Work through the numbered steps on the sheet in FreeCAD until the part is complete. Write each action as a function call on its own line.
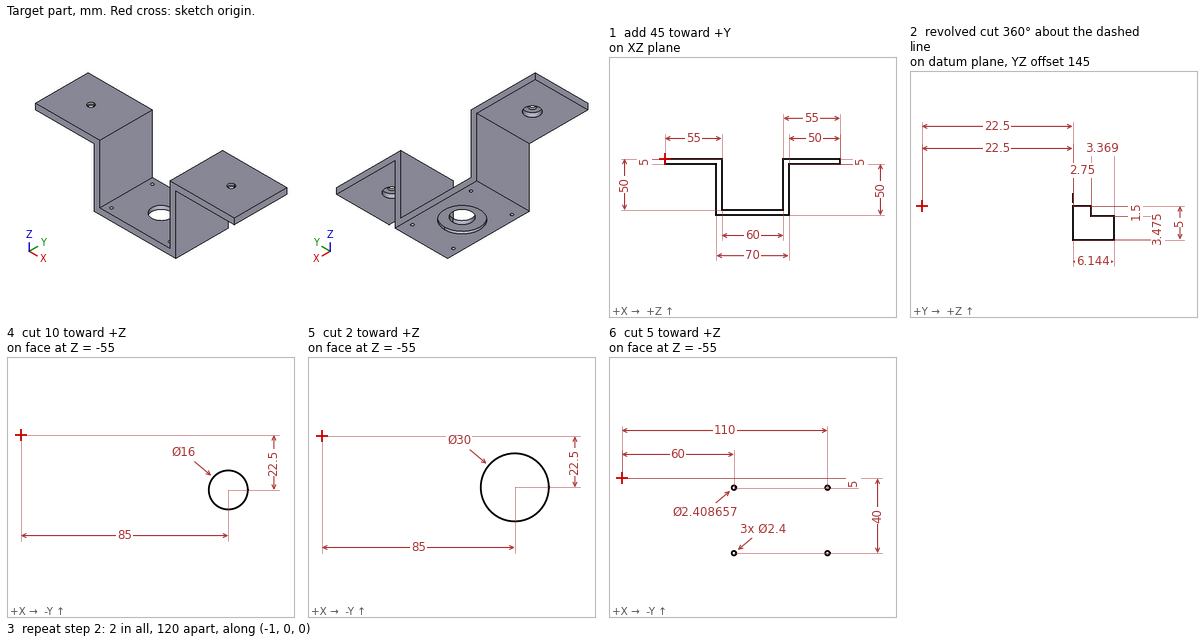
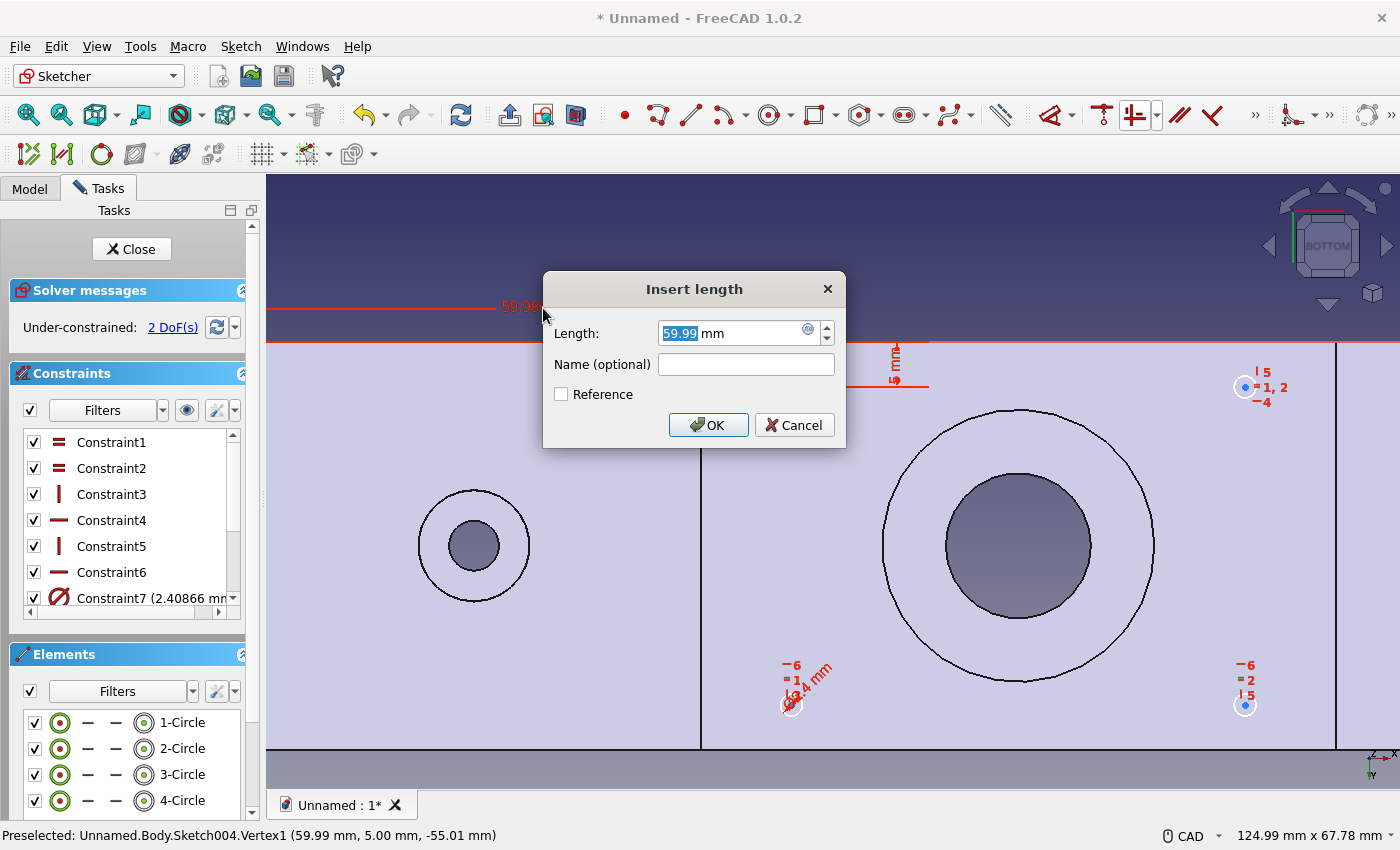
text(60)
key(Return)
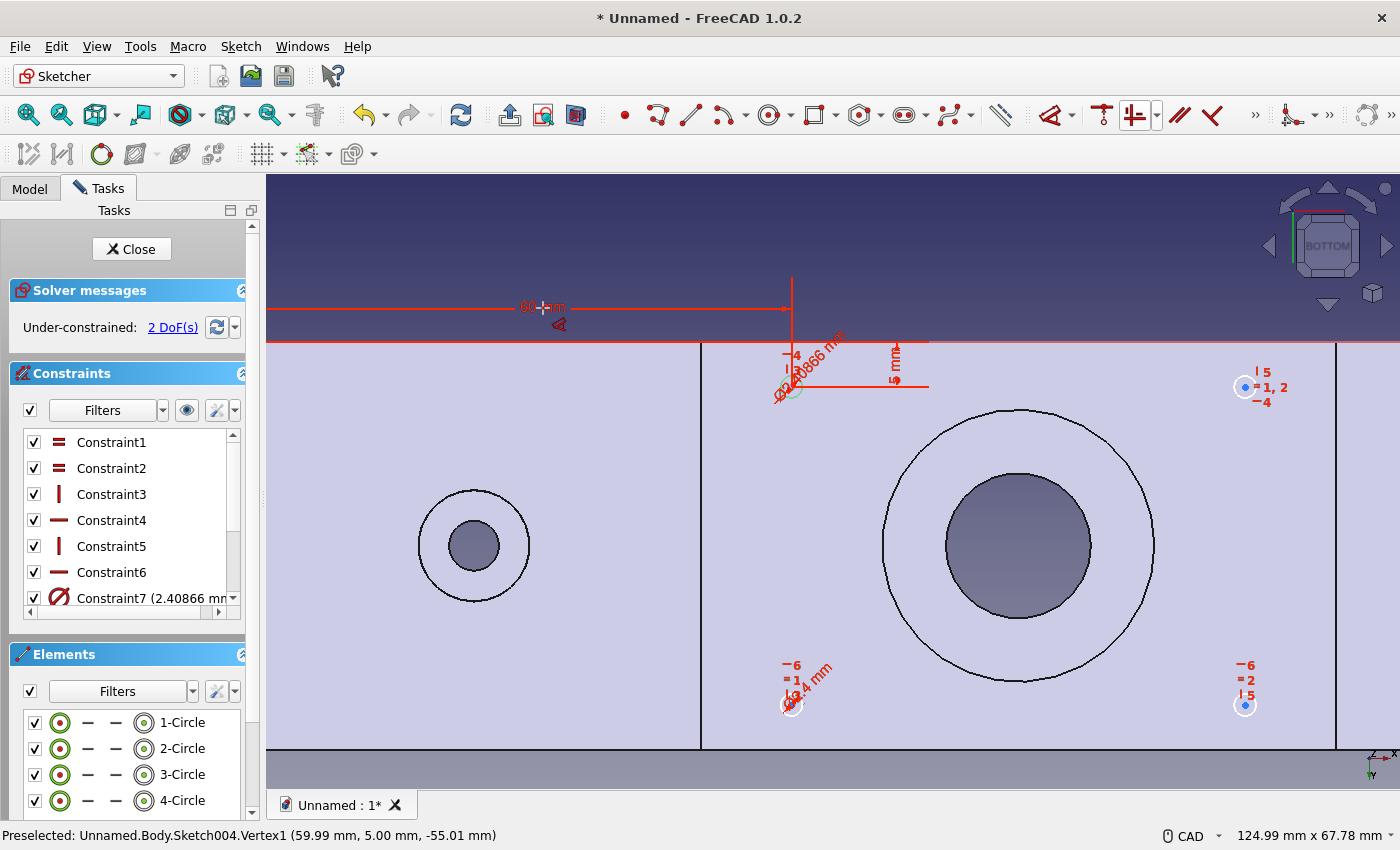
click(792, 705)
click(826, 523)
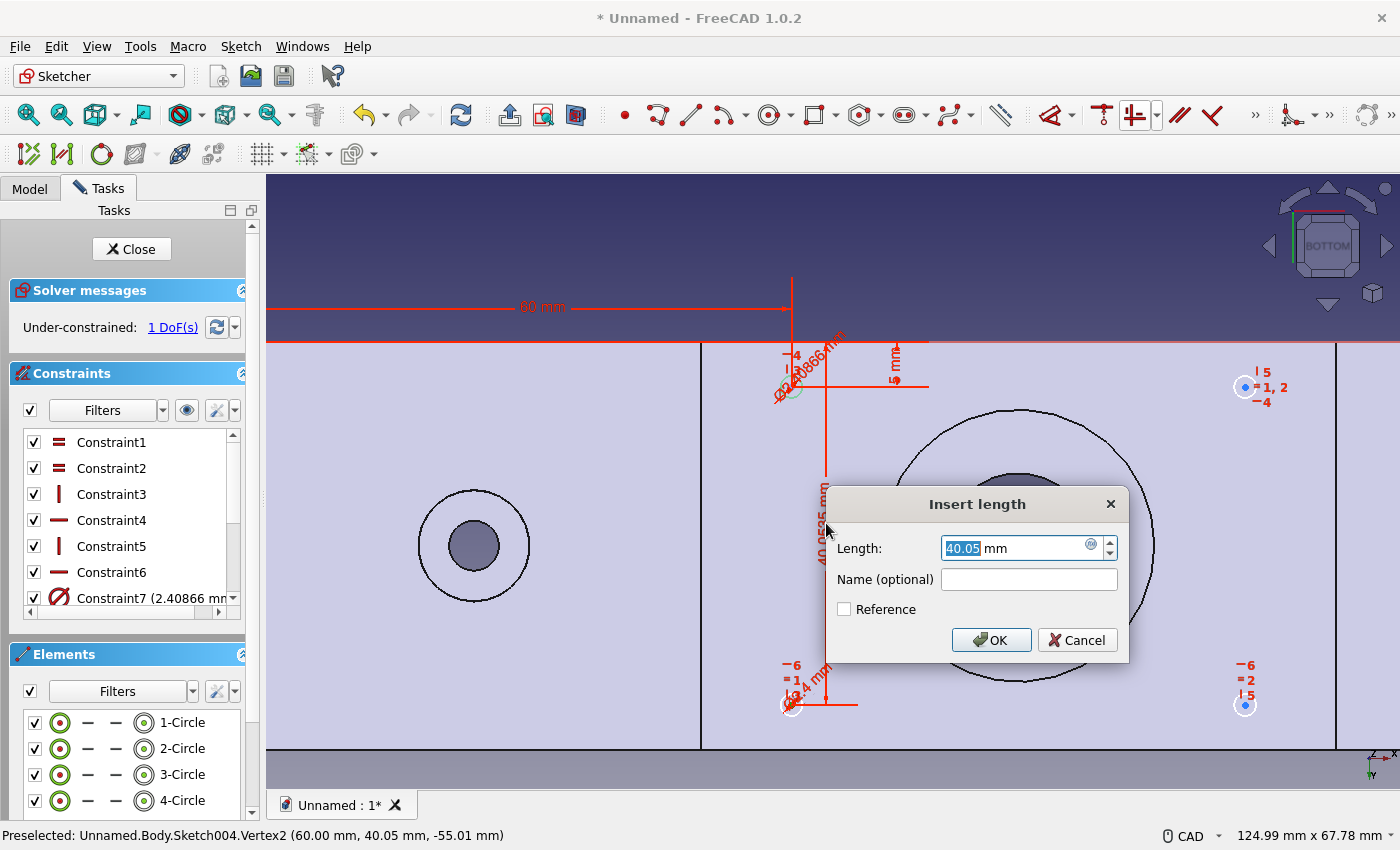
text(40)
key(Return)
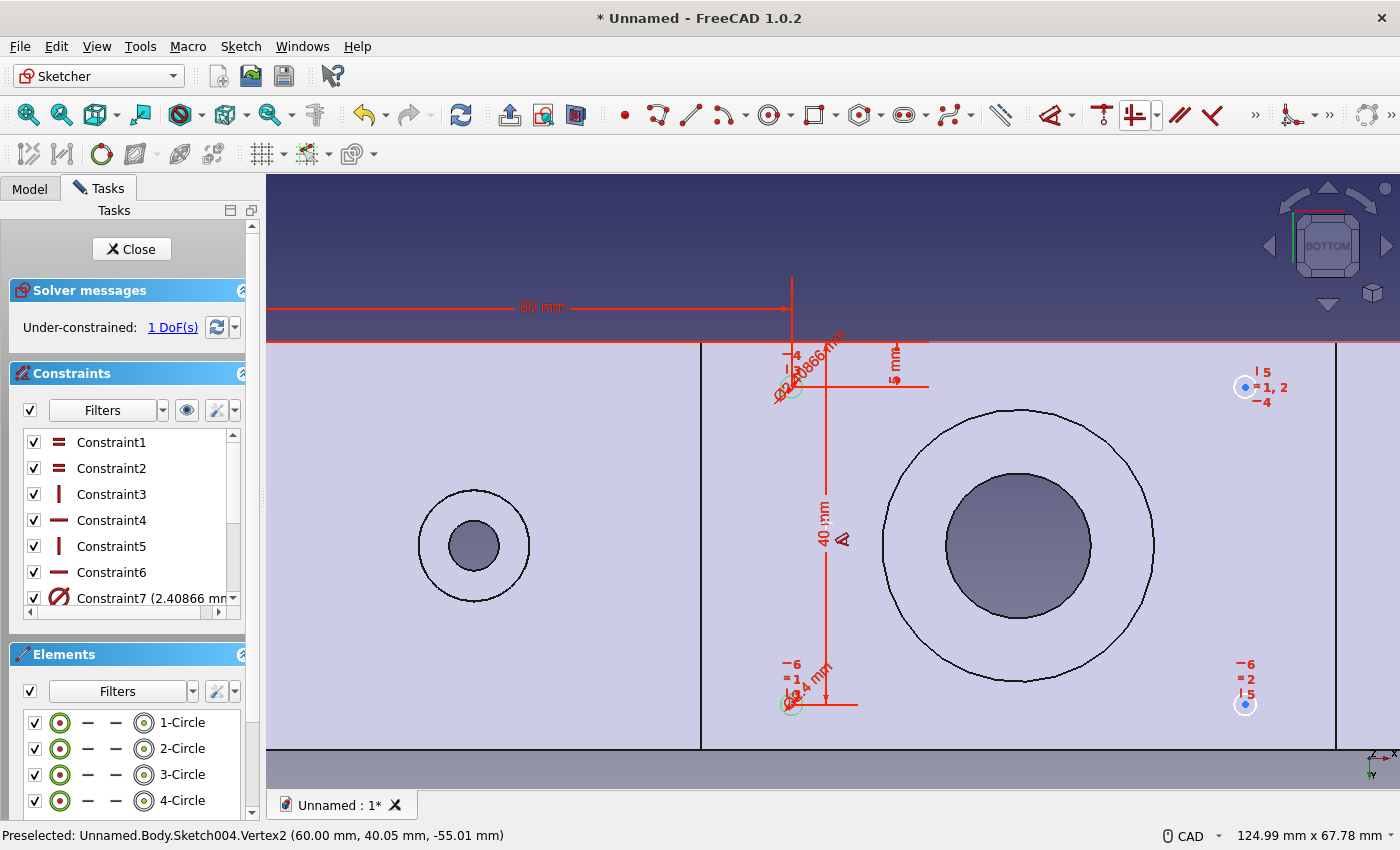
scroll(791, 386, down, 2)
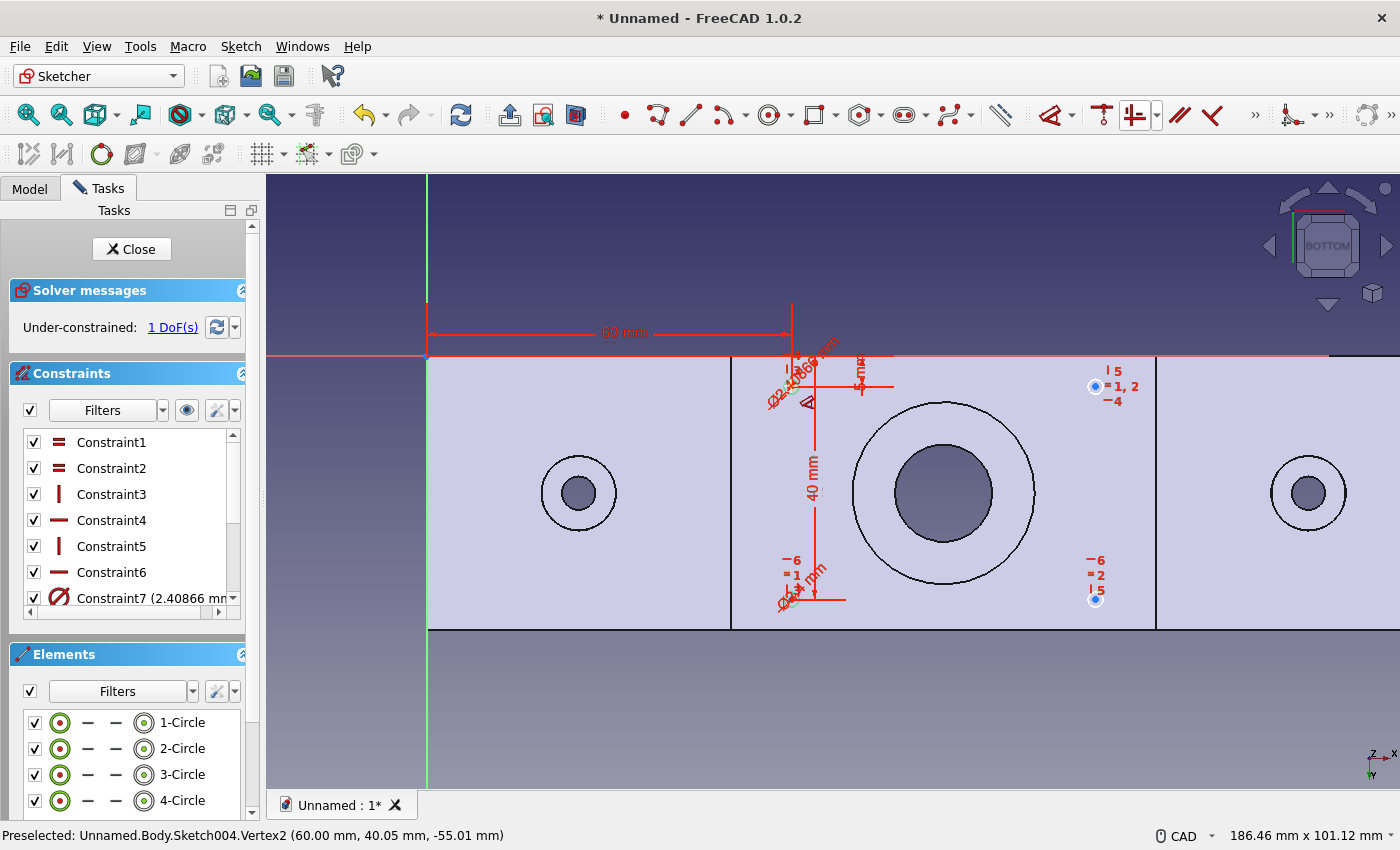
click(1096, 387)
click(761, 322)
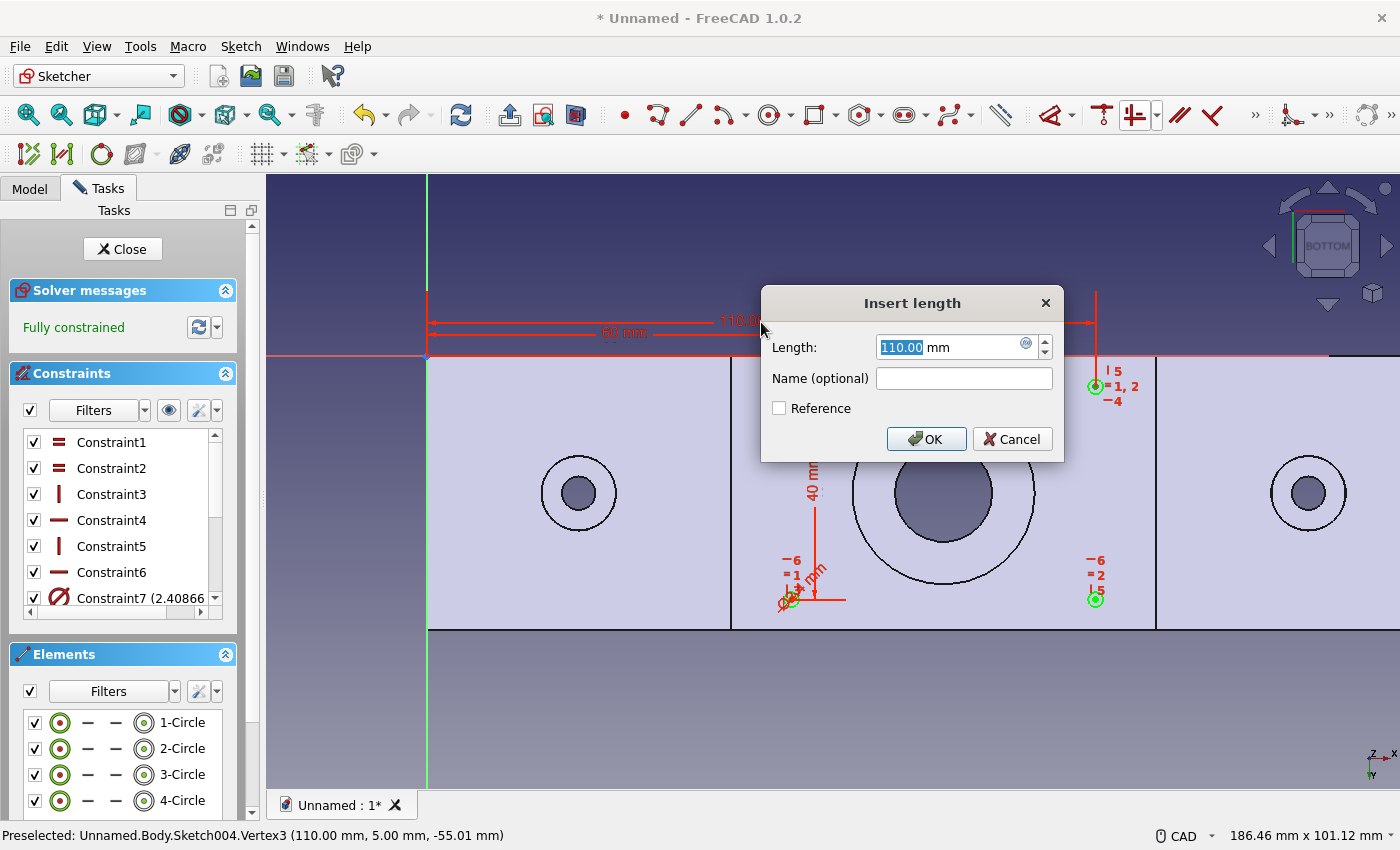
text(110)
key(Return)
key(Escape)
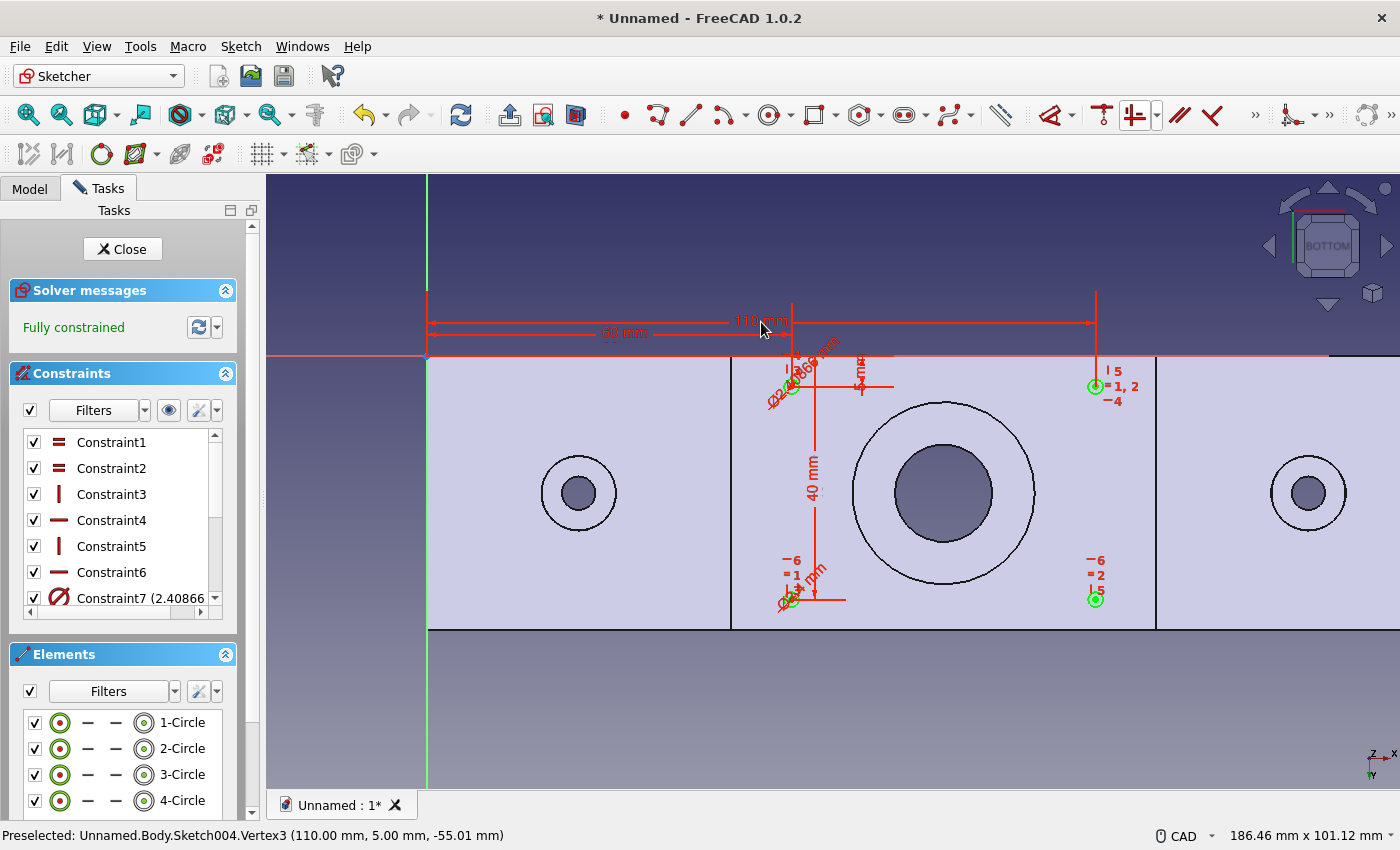
click(123, 249)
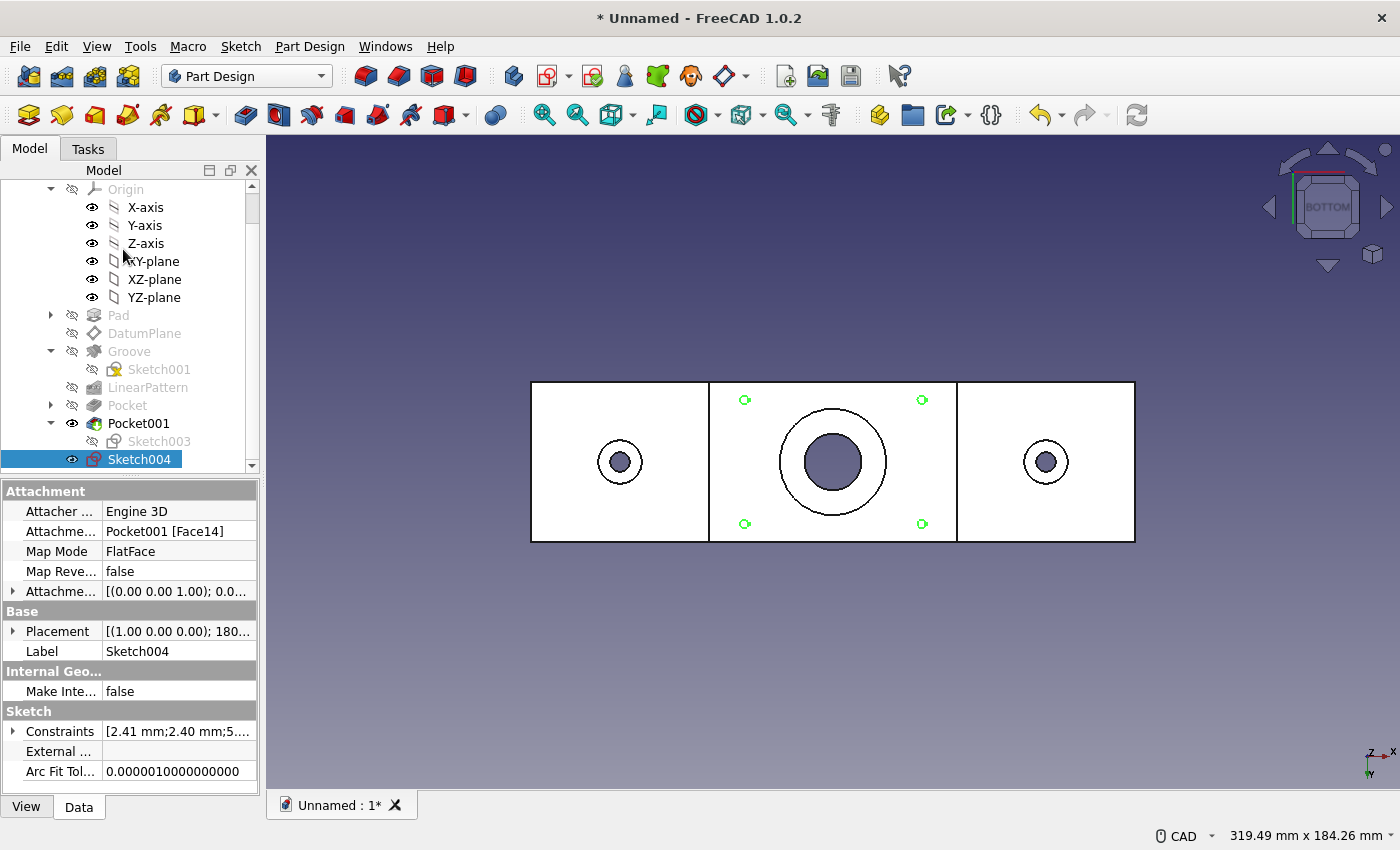
click(246, 116)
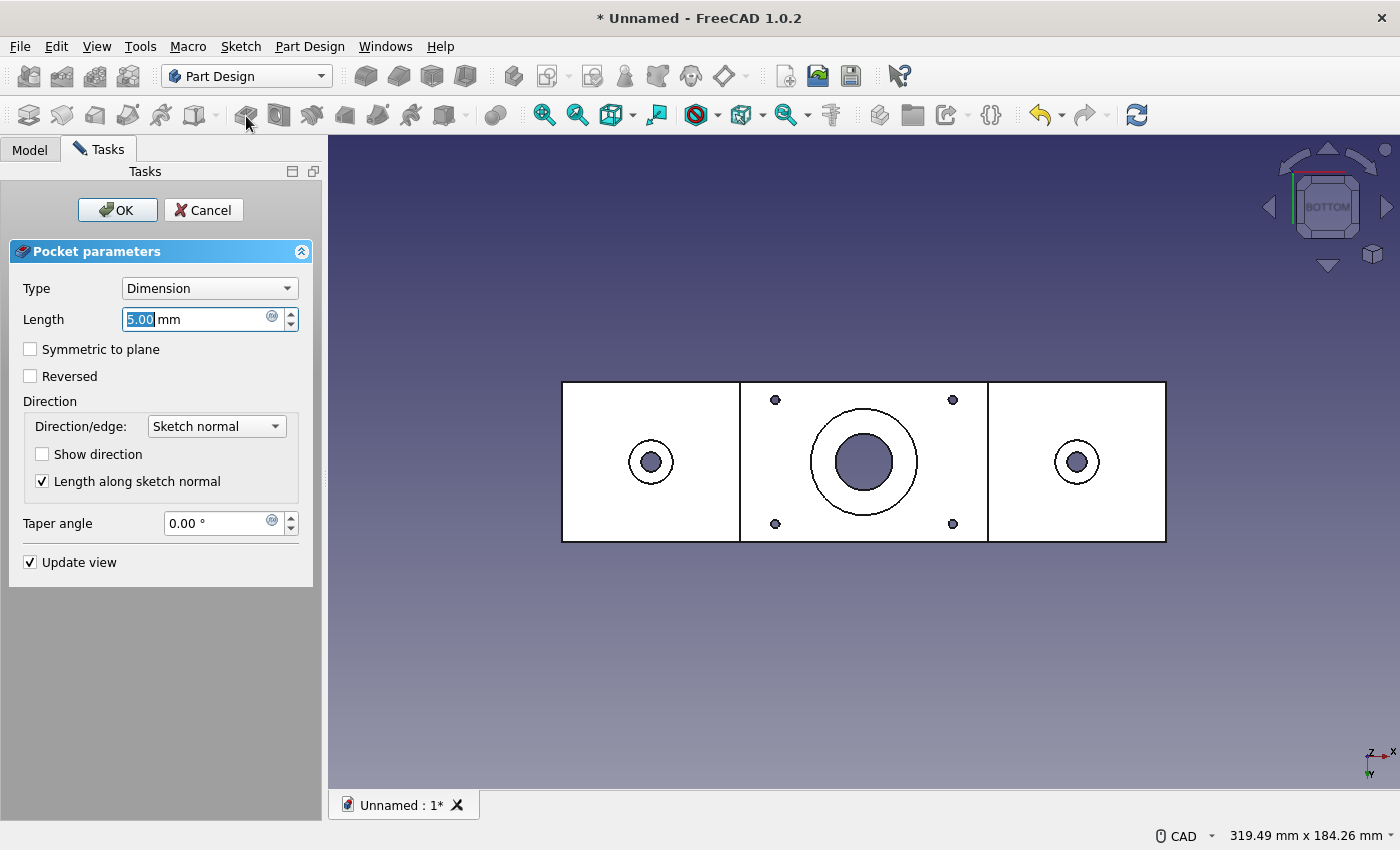
text(5)
key(Tab)